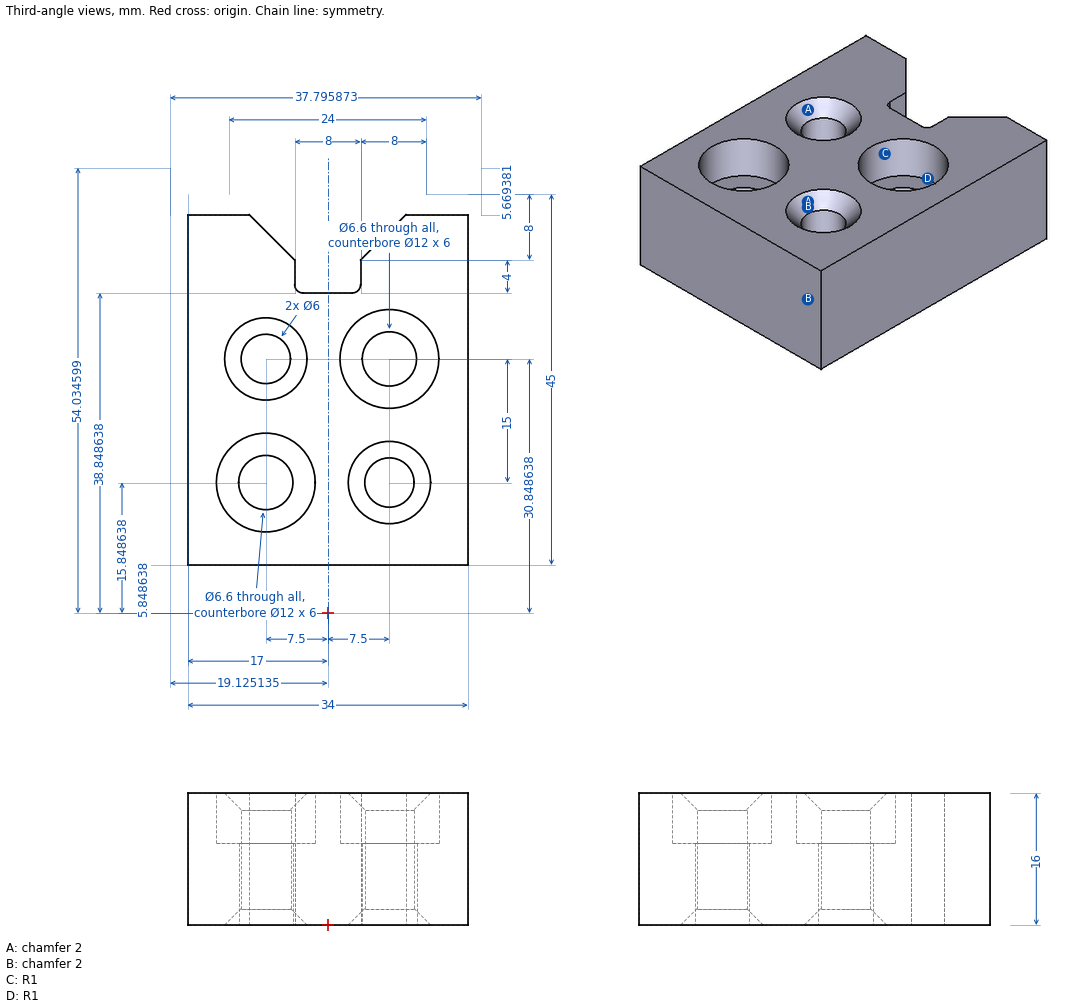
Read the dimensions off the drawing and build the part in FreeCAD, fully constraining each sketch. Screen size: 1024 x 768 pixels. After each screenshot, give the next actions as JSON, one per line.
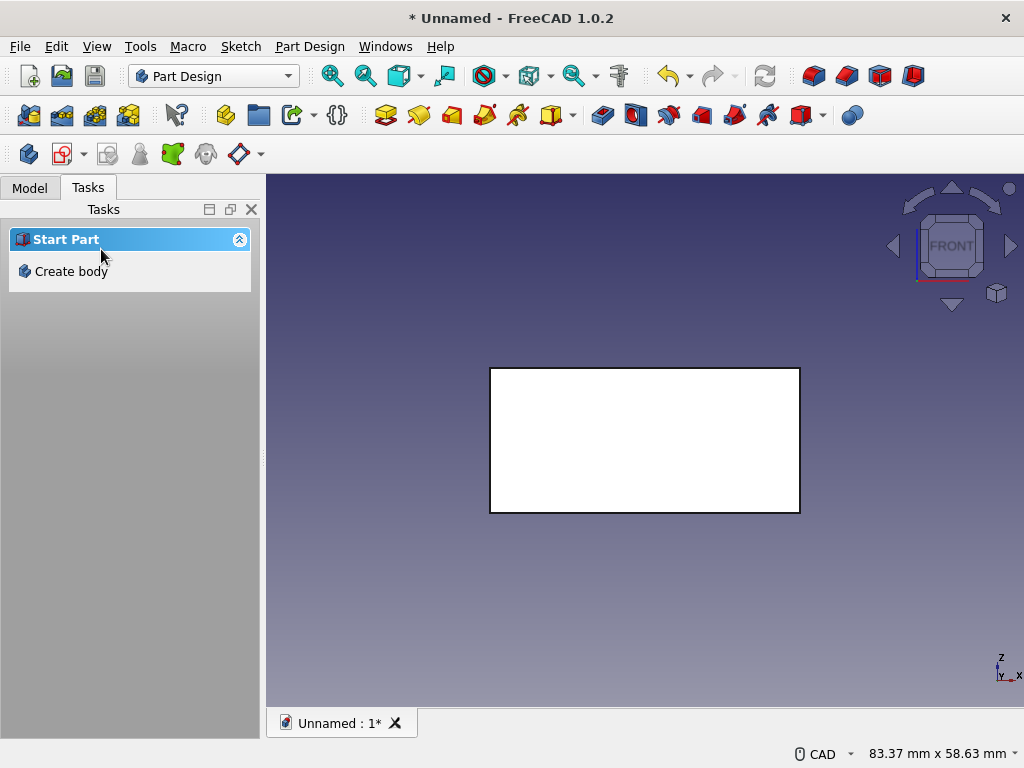
{"action": "left_click", "coordinate": [333, 76]}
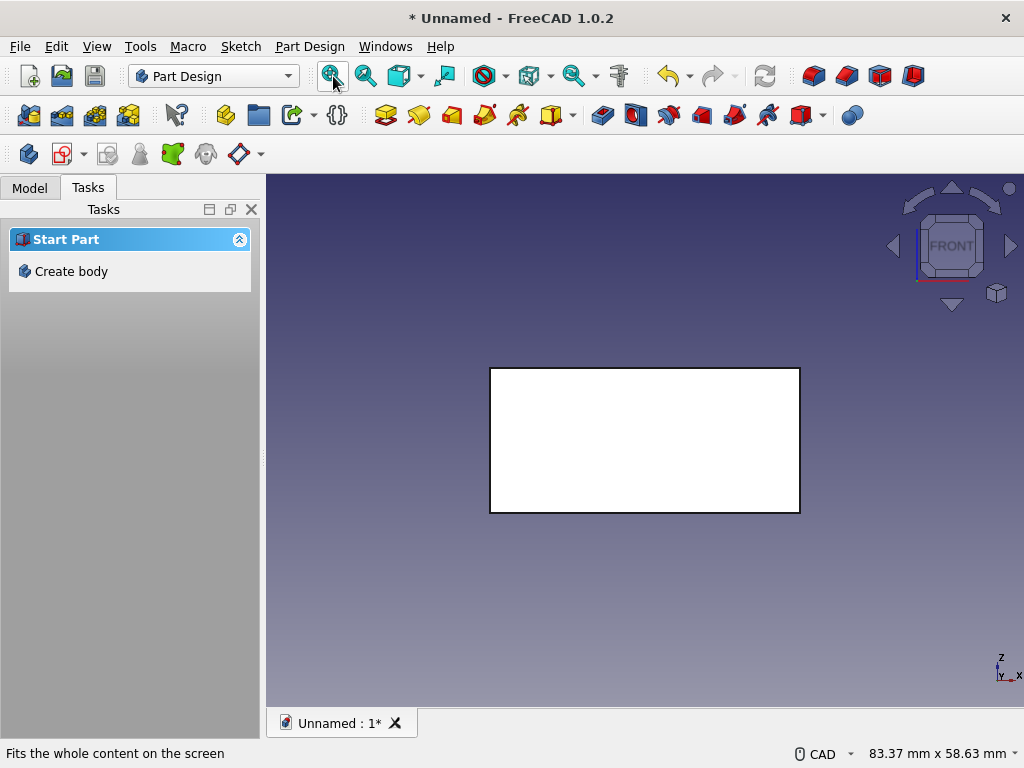
{"action": "key", "text": "3"}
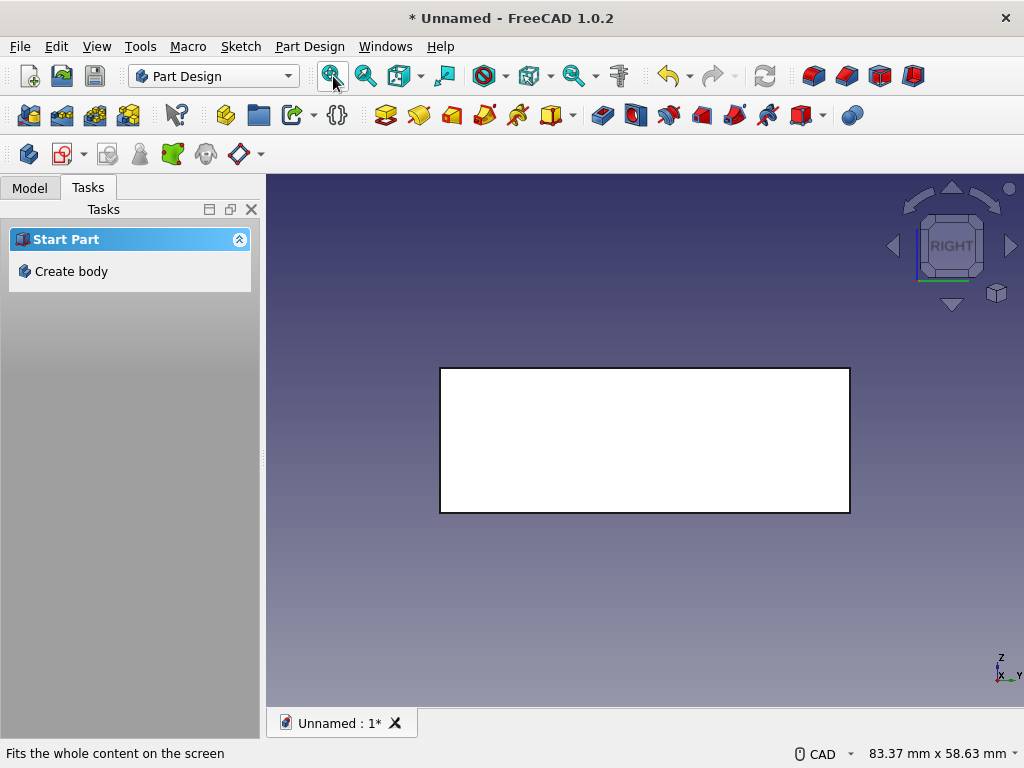
{"action": "key", "text": "5"}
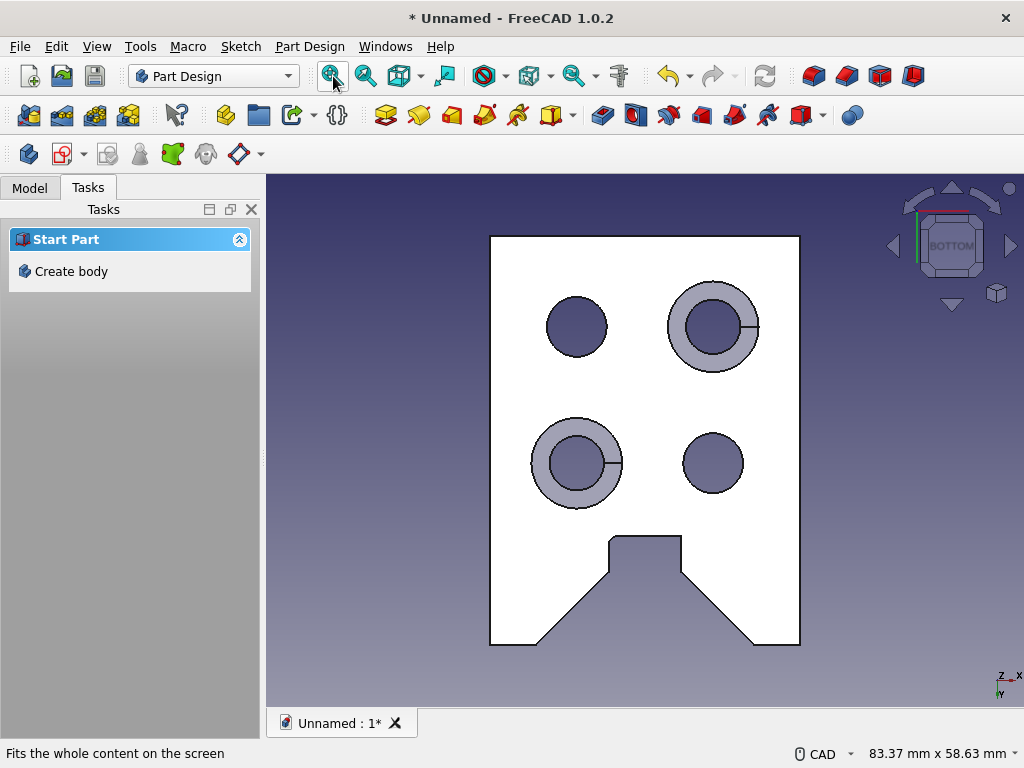
{"action": "key", "text": "4"}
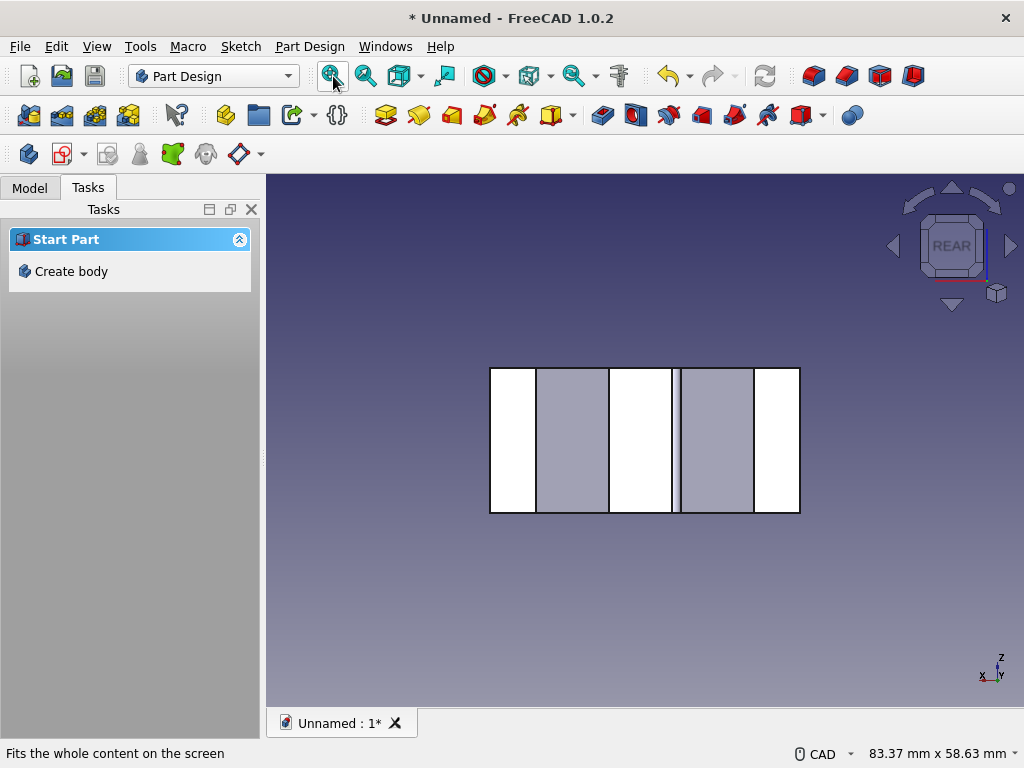
{"action": "key", "text": "v f"}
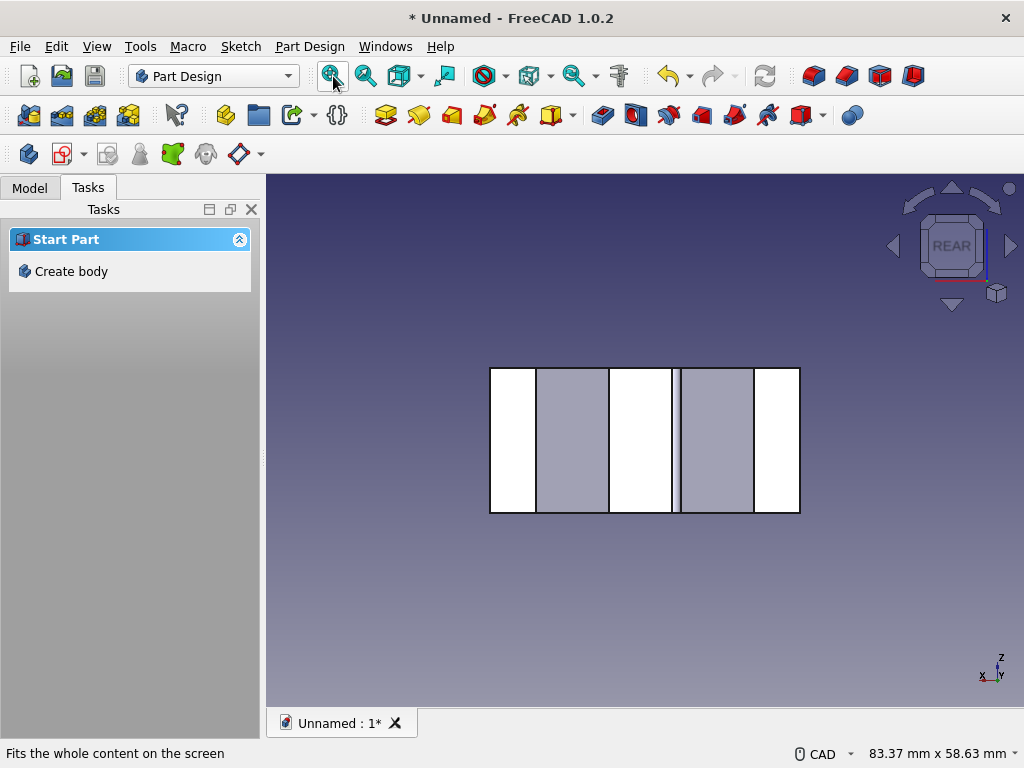
{"action": "key", "text": "6"}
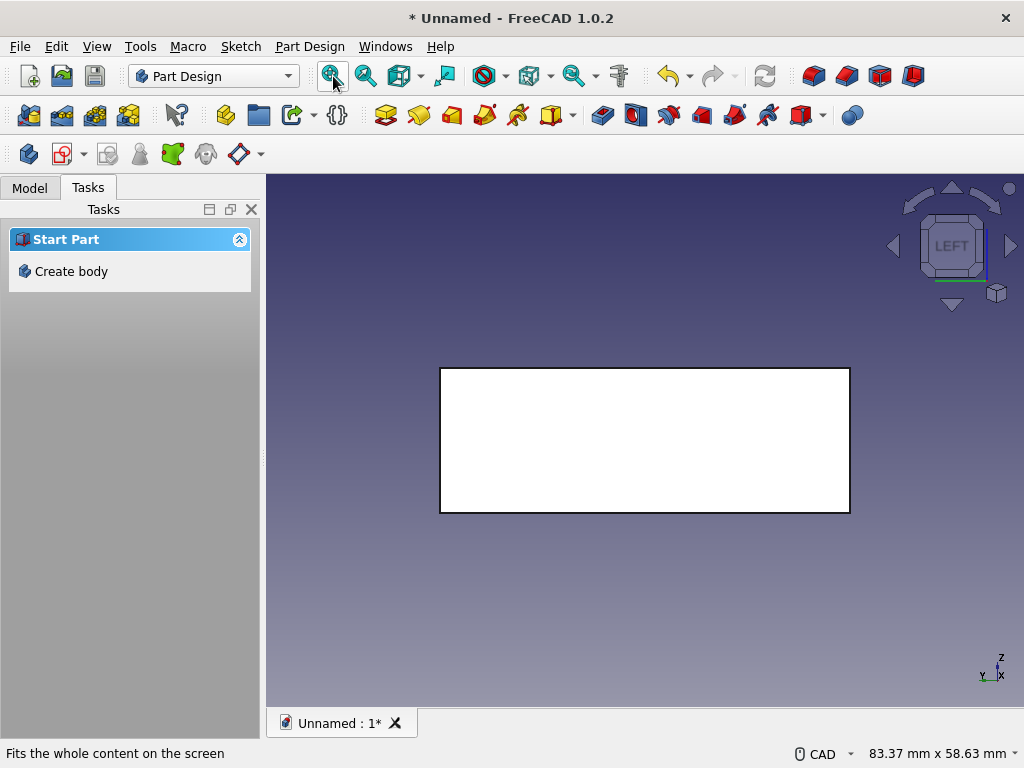
{"action": "key", "text": "v 3"}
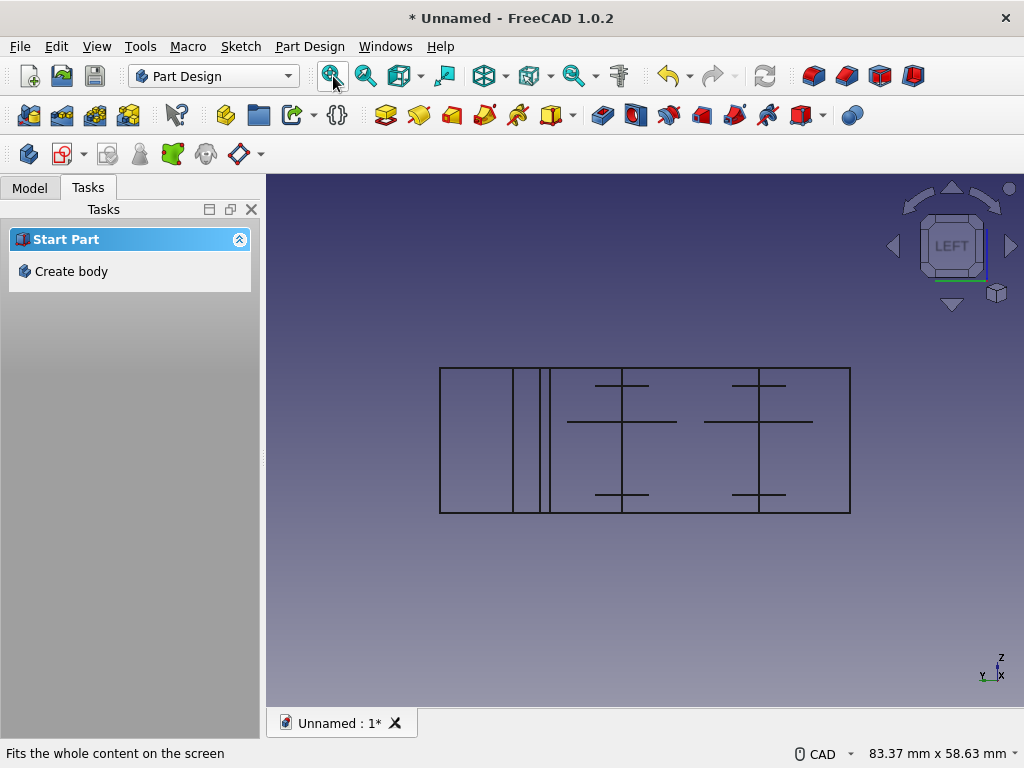
{"action": "key", "text": "0"}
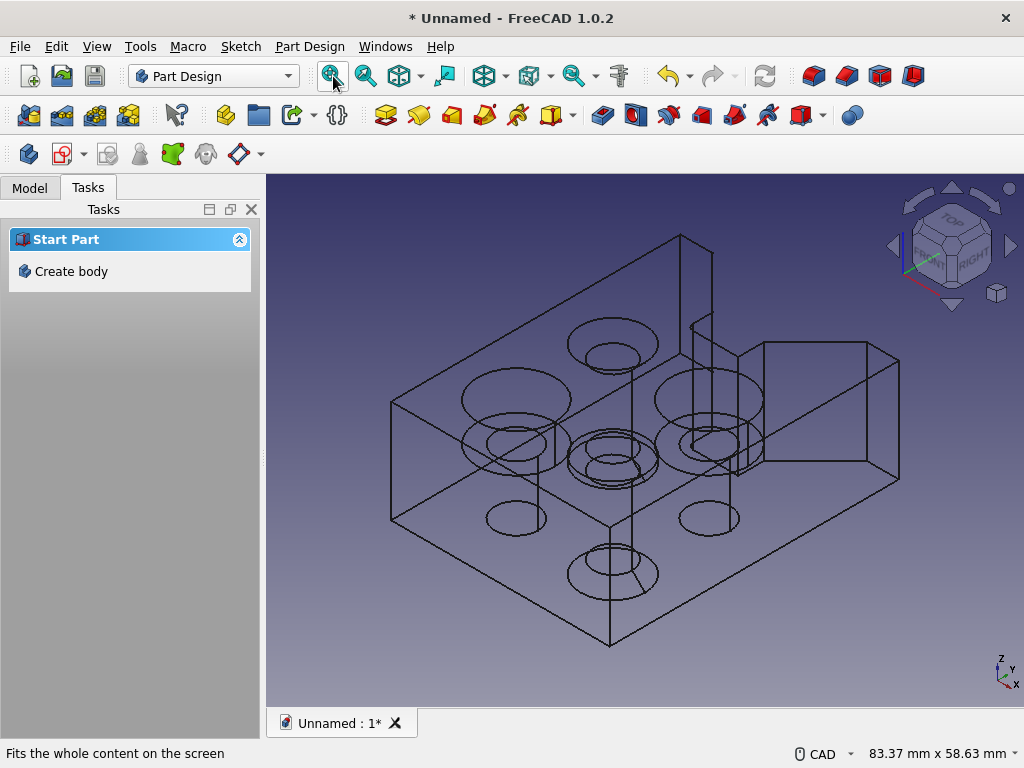
{"action": "left_click", "coordinate": [738, 403]}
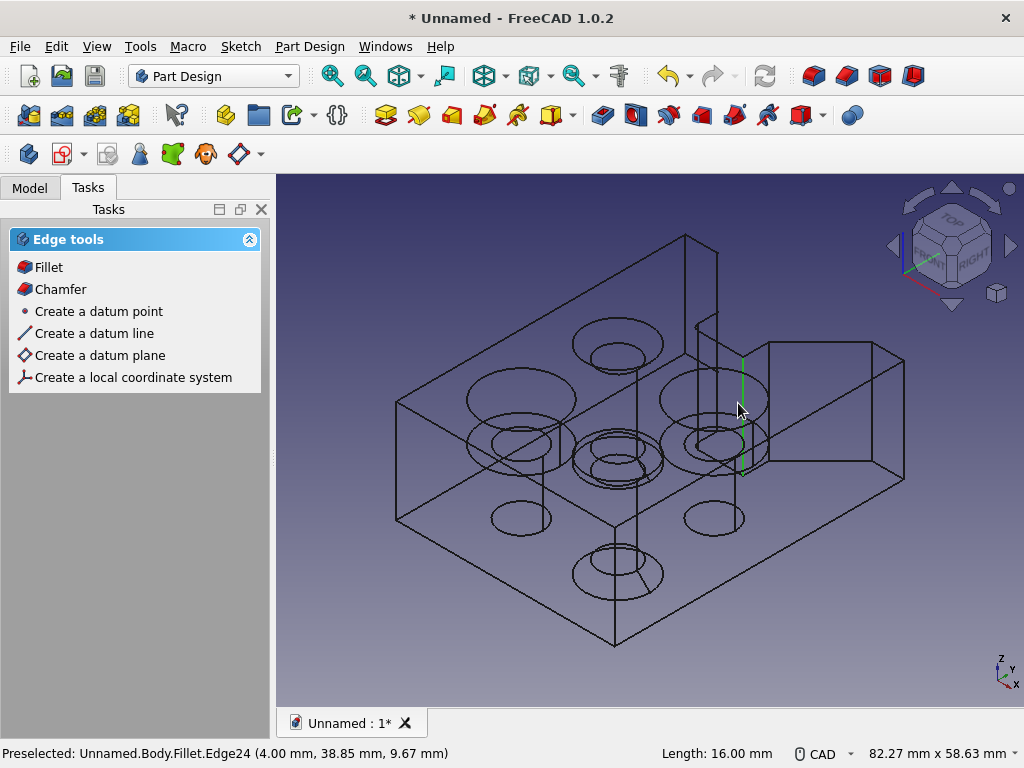
{"action": "key", "text": "v 1"}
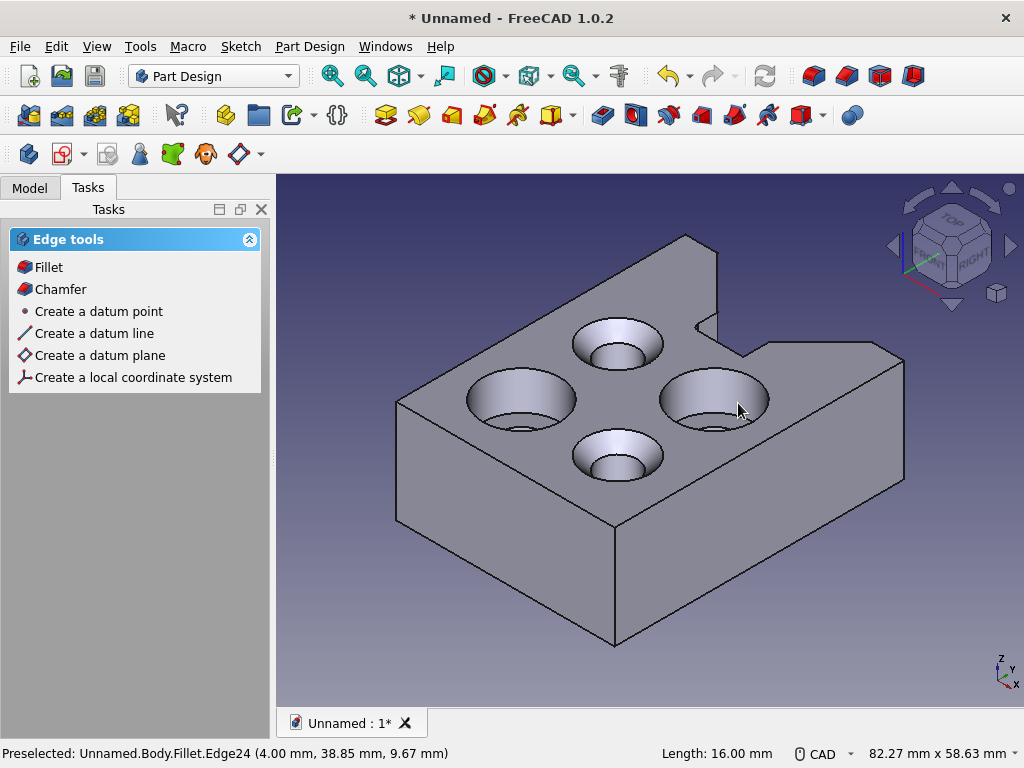
{"action": "left_click", "coordinate": [814, 76]}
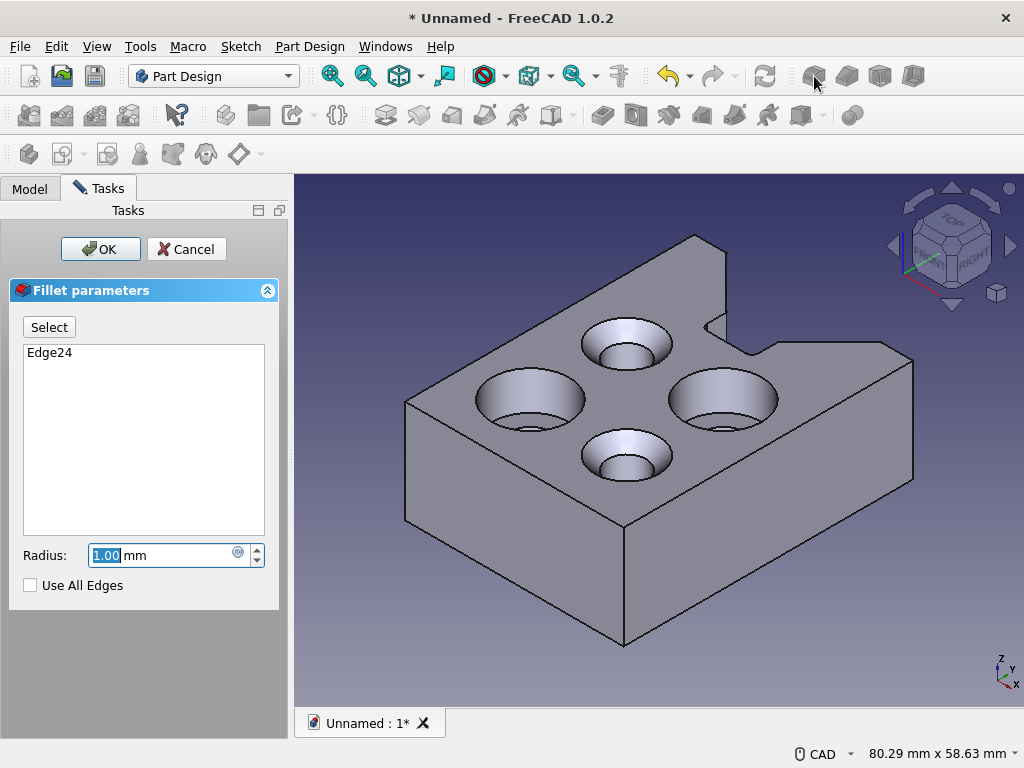
{"action": "type", "text": "1"}
{"action": "key", "text": "Tab"}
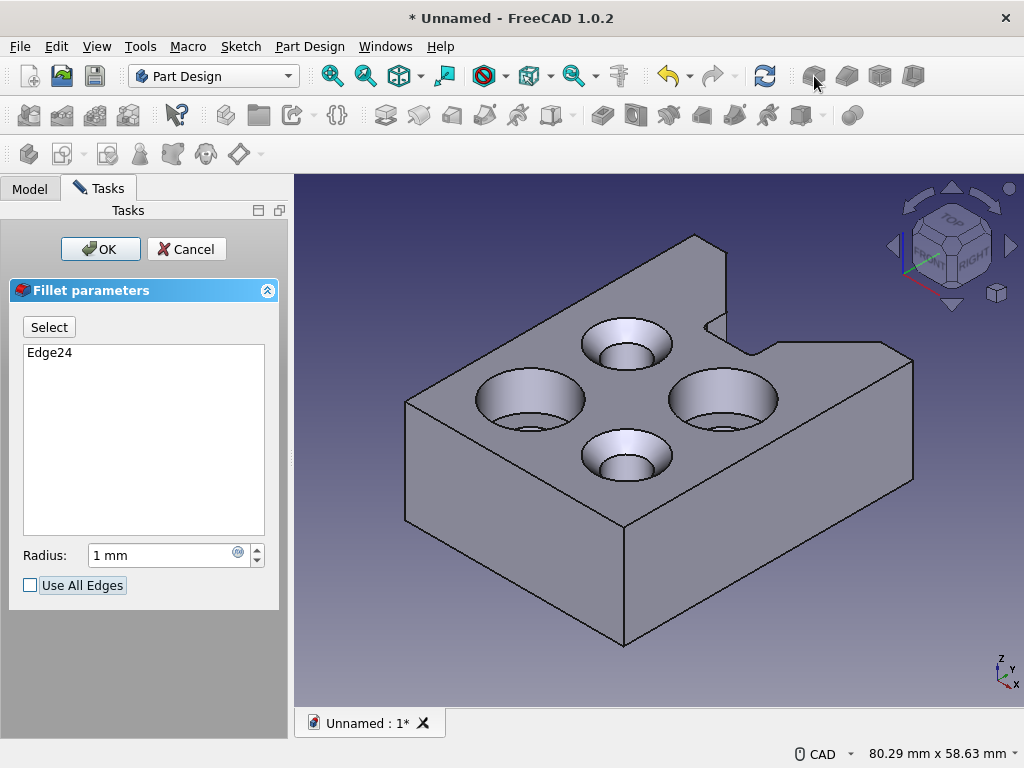
{"action": "left_click", "coordinate": [101, 249]}